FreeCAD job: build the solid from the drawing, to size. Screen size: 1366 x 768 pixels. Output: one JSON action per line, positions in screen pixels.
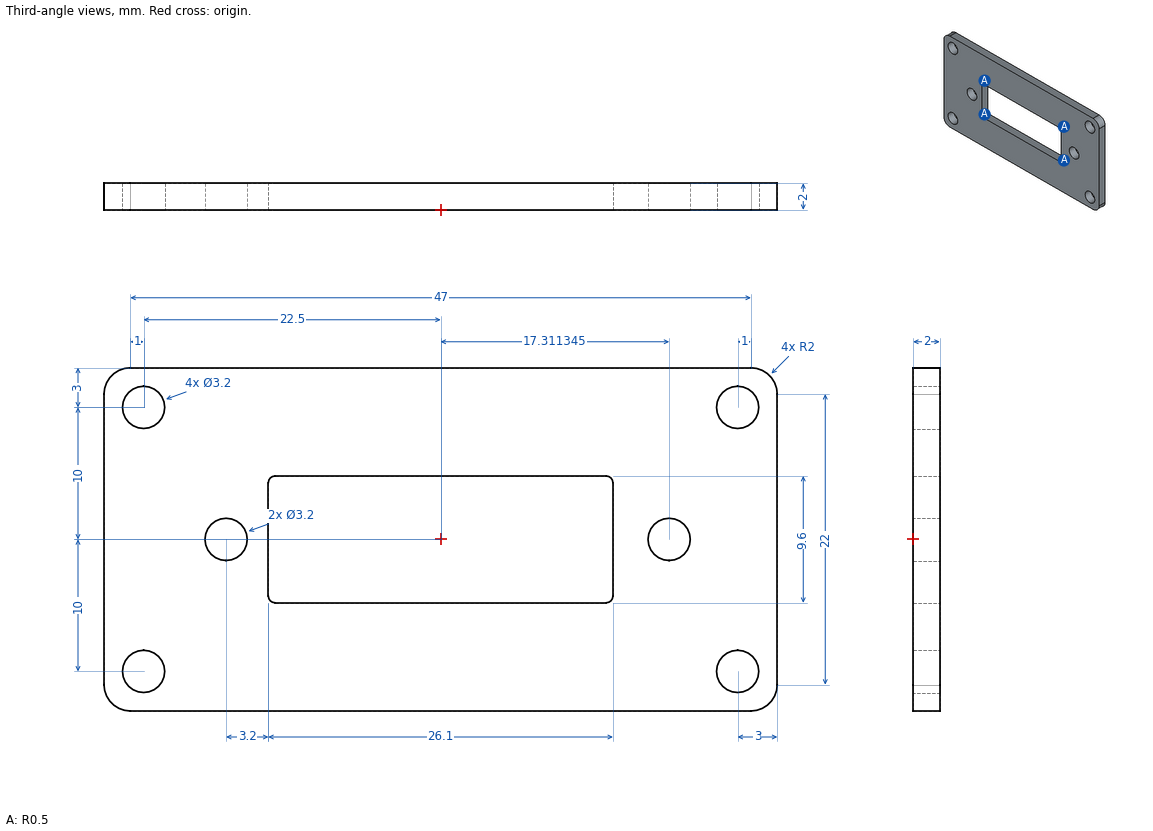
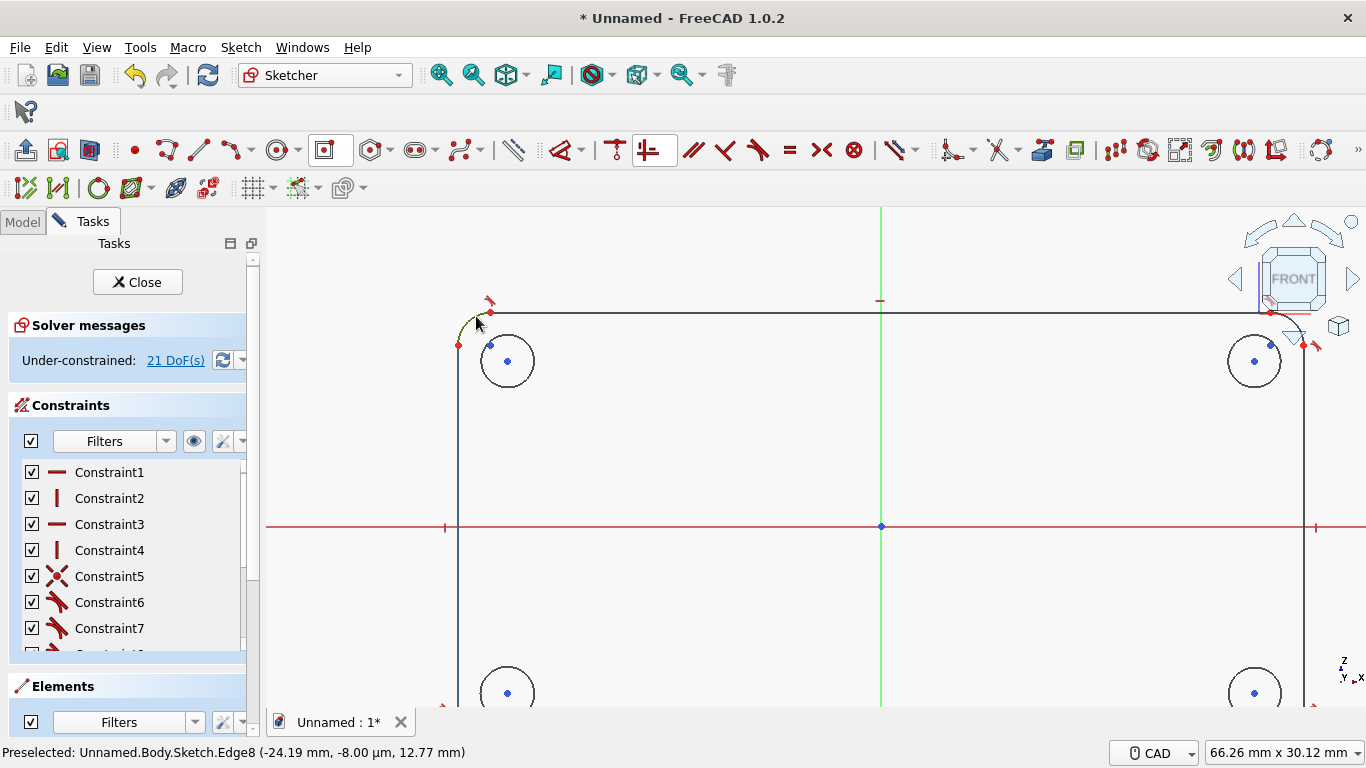
{"action": "left_click", "coordinate": [758, 150]}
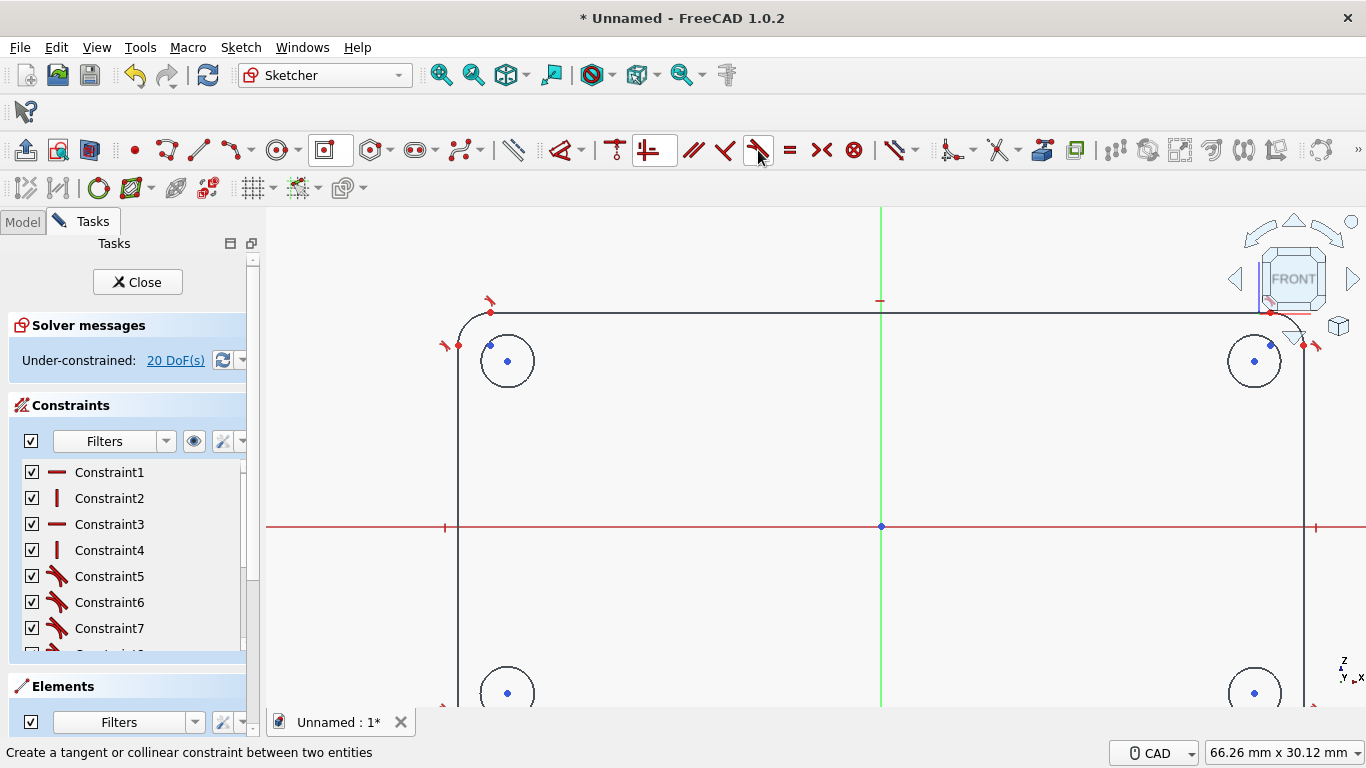
{"action": "scroll", "coordinate": [476, 315], "scroll_direction": "down", "scroll_amount": 2}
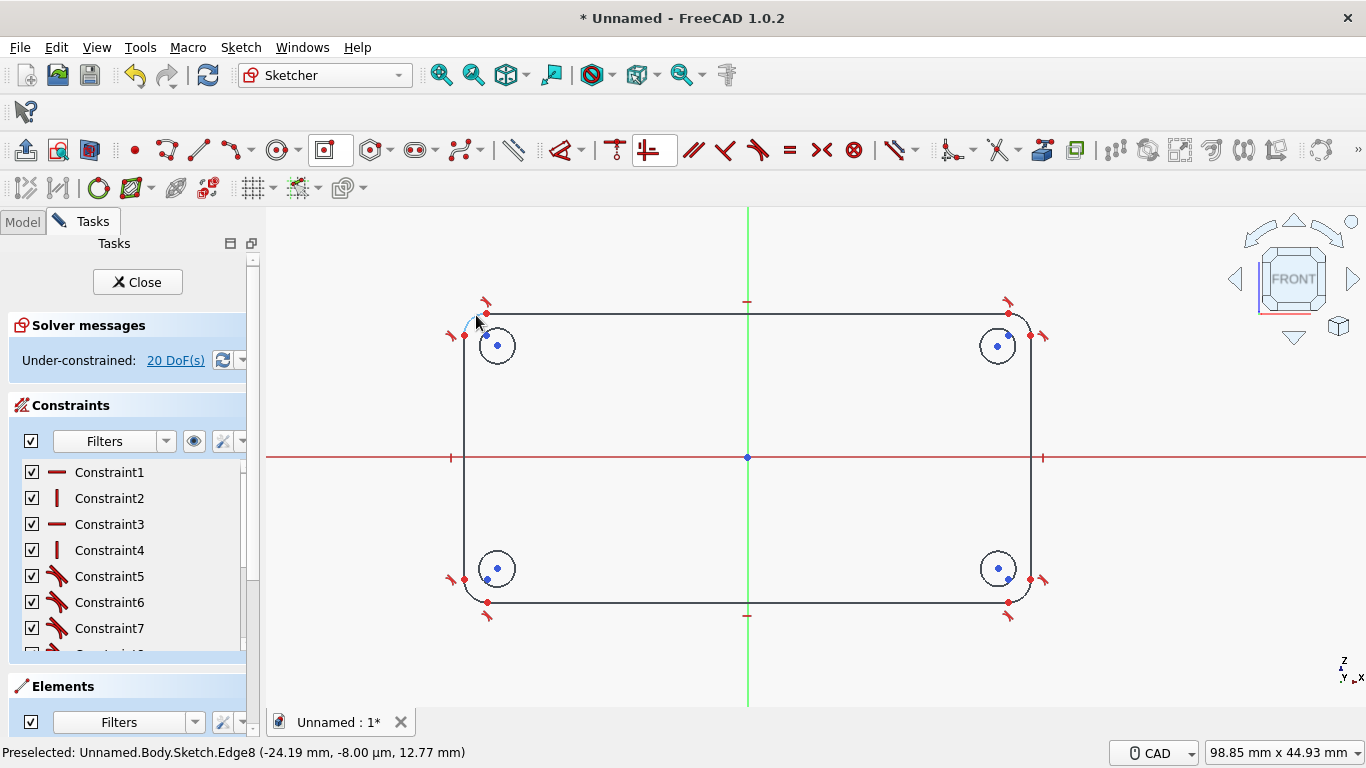
{"action": "scroll", "coordinate": [1029, 326], "scroll_direction": "up", "scroll_amount": 2}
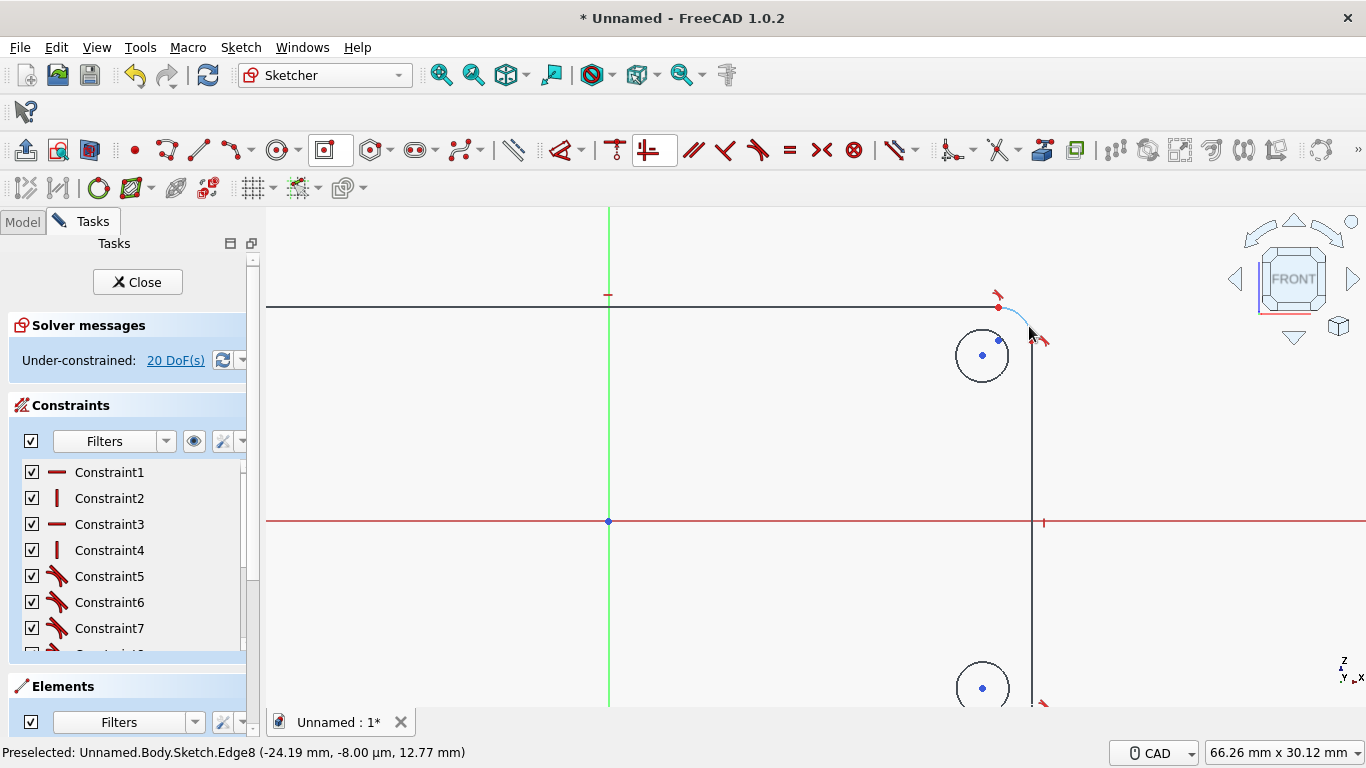
{"action": "left_click", "coordinate": [1028, 325]}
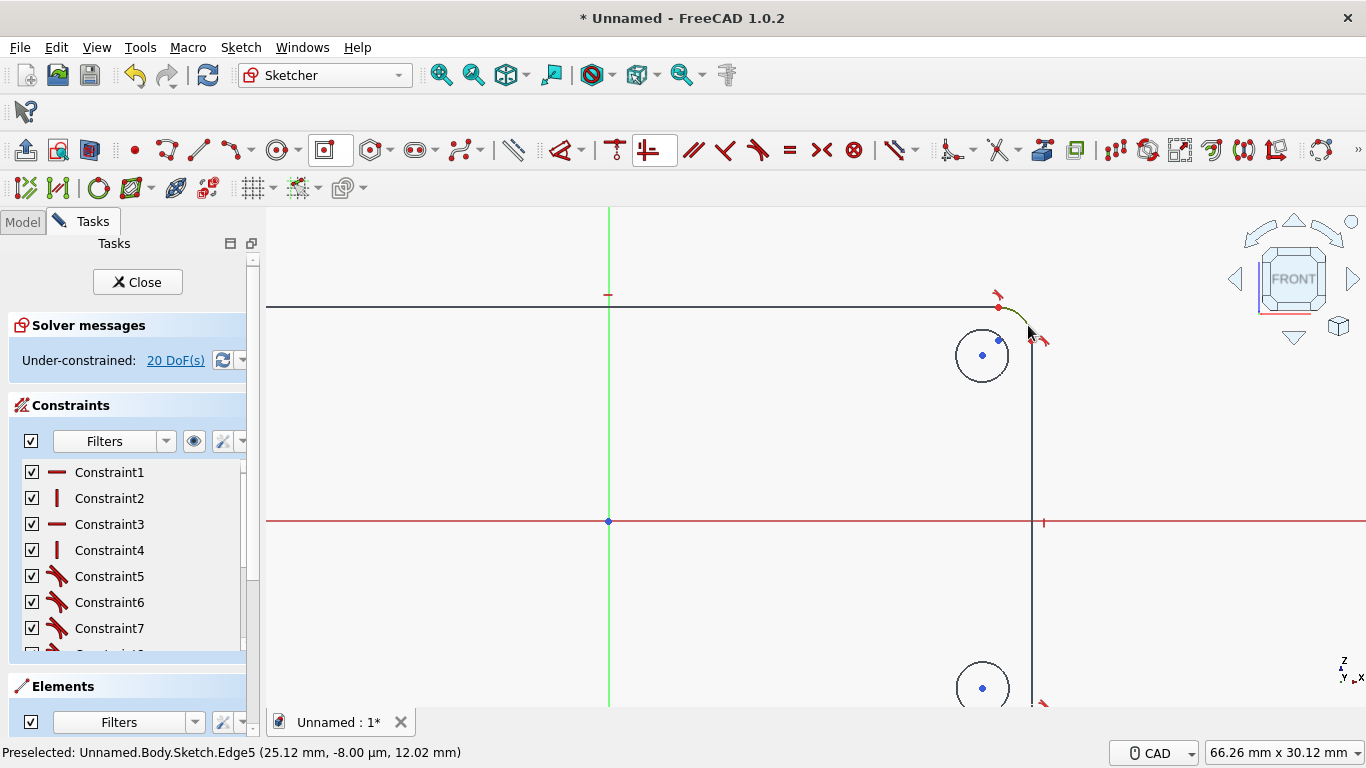
{"action": "scroll", "coordinate": [1029, 326], "scroll_direction": "down", "scroll_amount": 2}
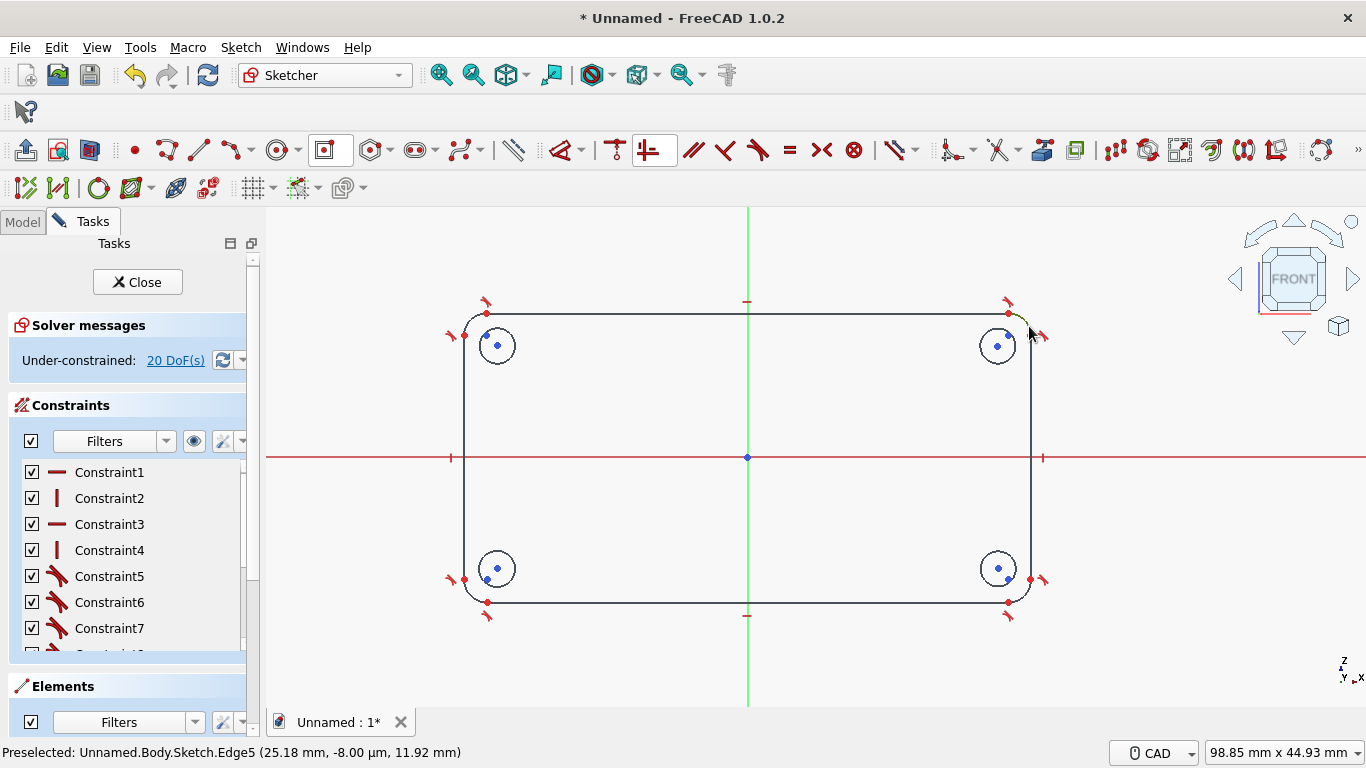
{"action": "scroll", "coordinate": [1019, 600], "scroll_direction": "up", "scroll_amount": 2}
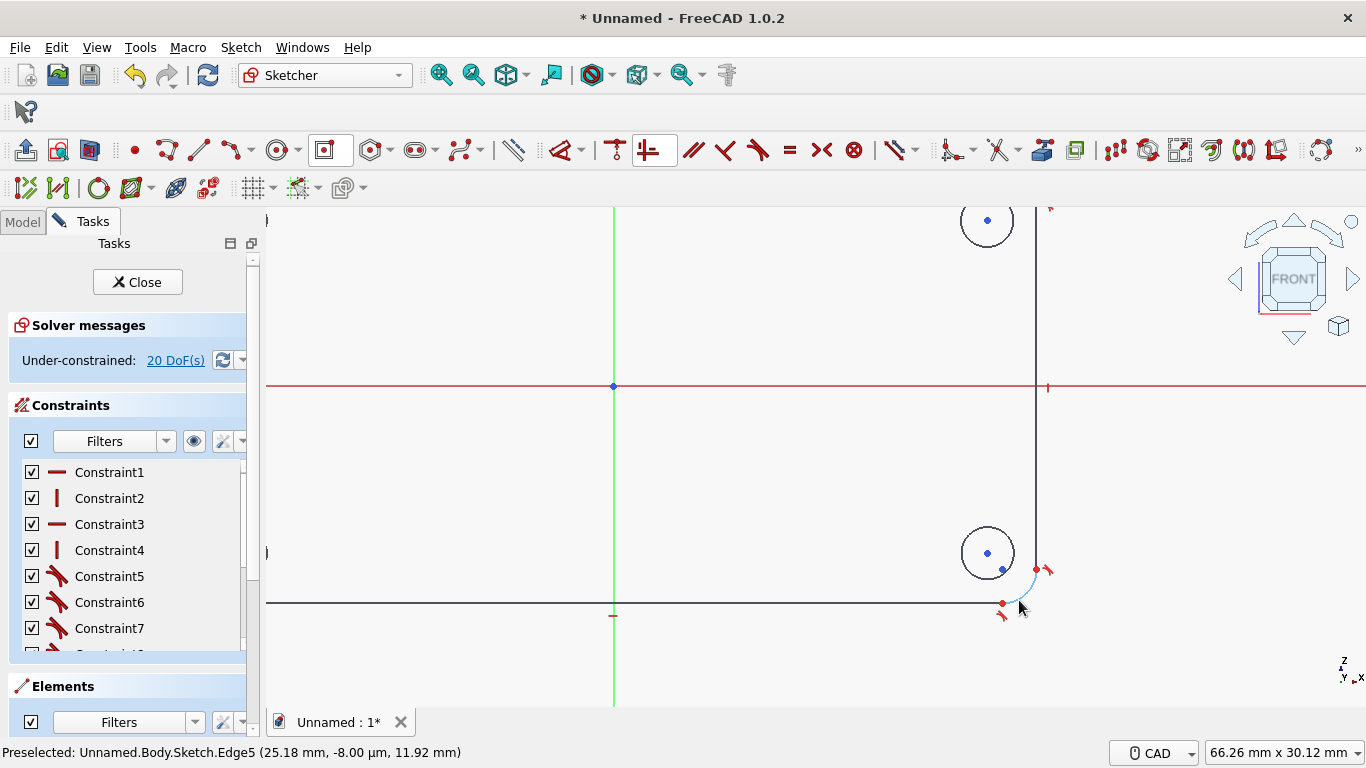
{"action": "left_click", "coordinate": [1018, 600]}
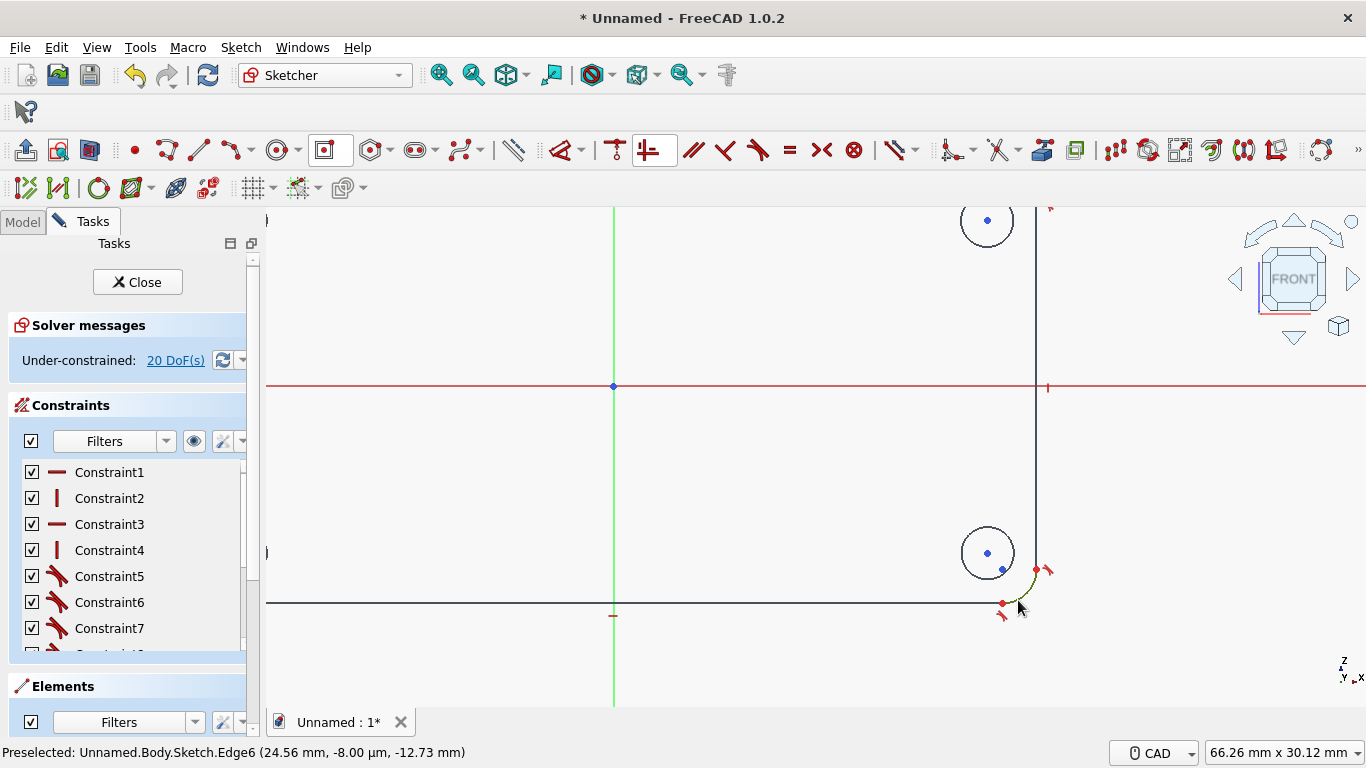
{"action": "scroll", "coordinate": [1019, 601], "scroll_direction": "down", "scroll_amount": 2}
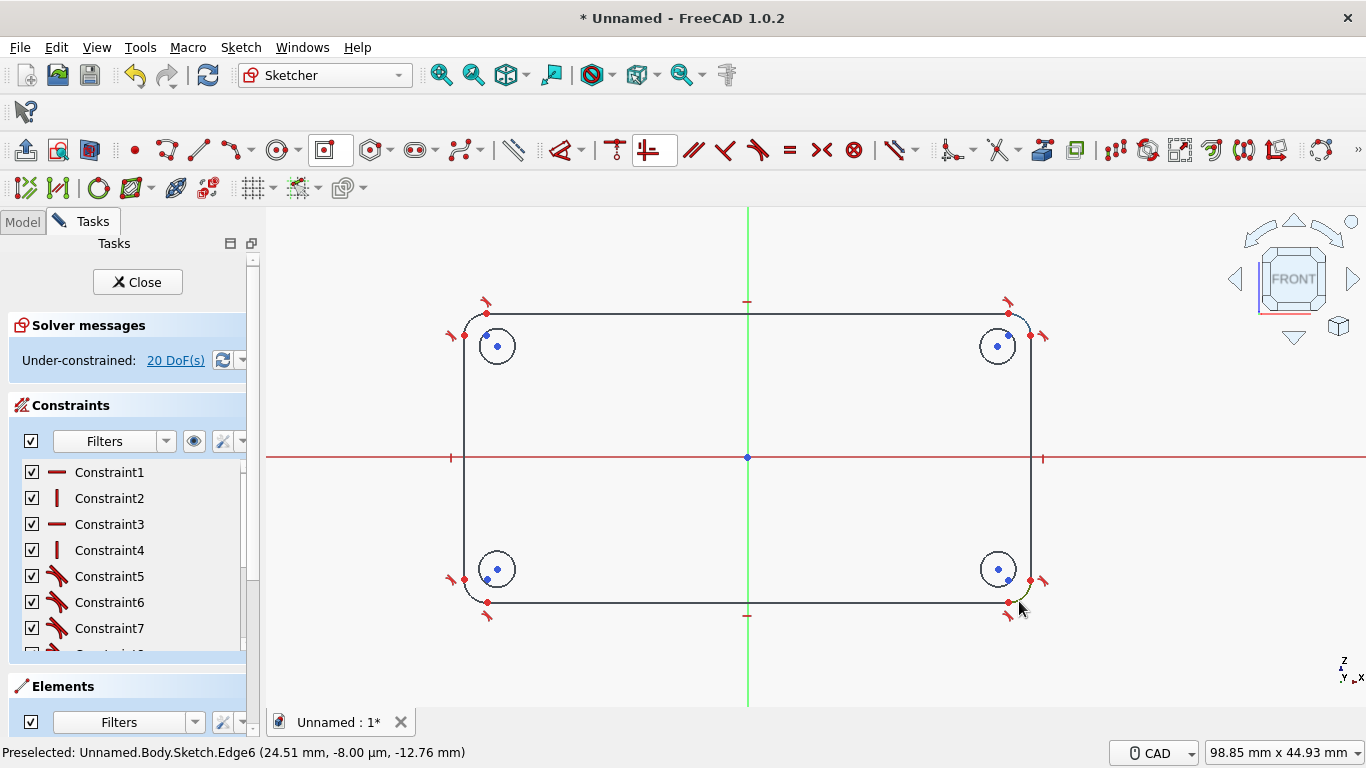
{"action": "scroll", "coordinate": [467, 590], "scroll_direction": "up", "scroll_amount": 2}